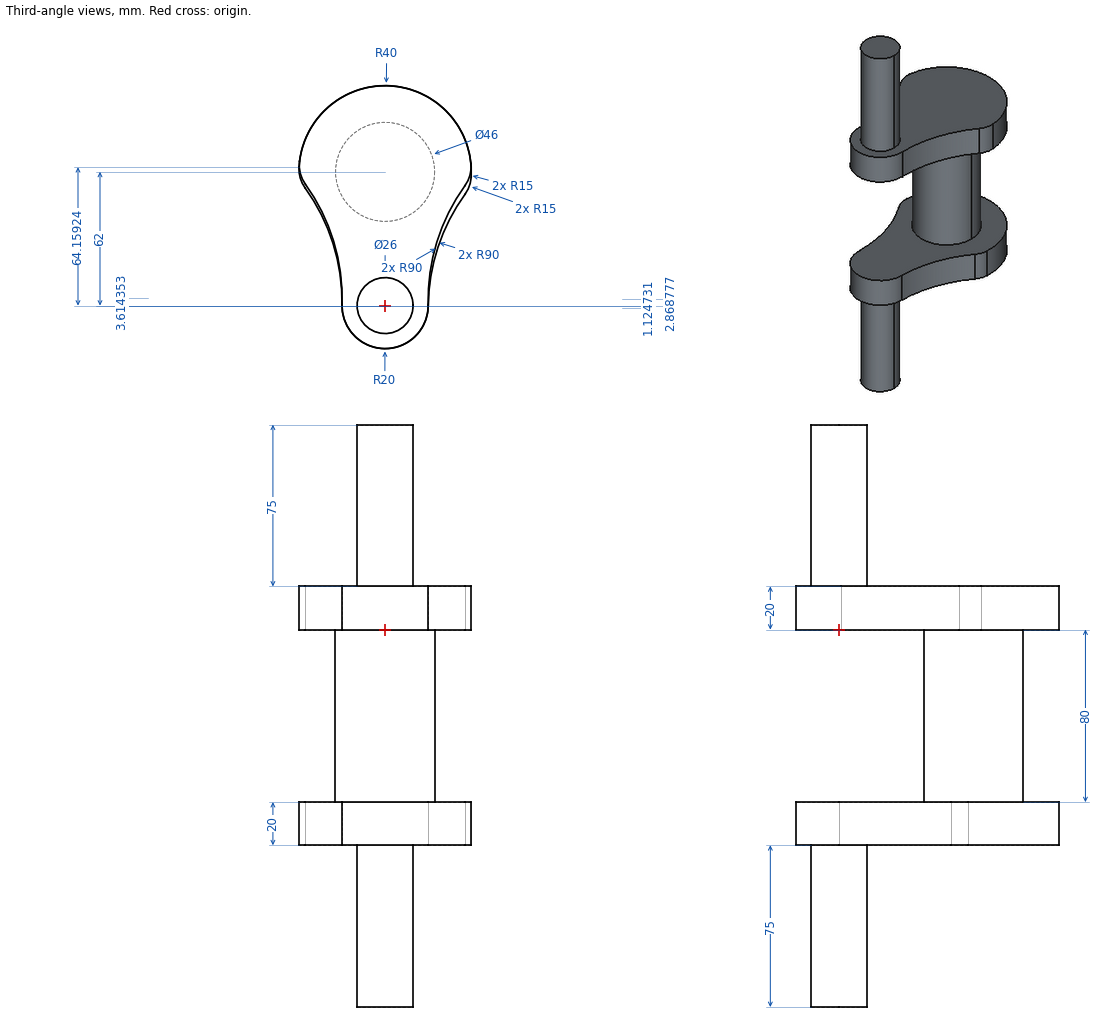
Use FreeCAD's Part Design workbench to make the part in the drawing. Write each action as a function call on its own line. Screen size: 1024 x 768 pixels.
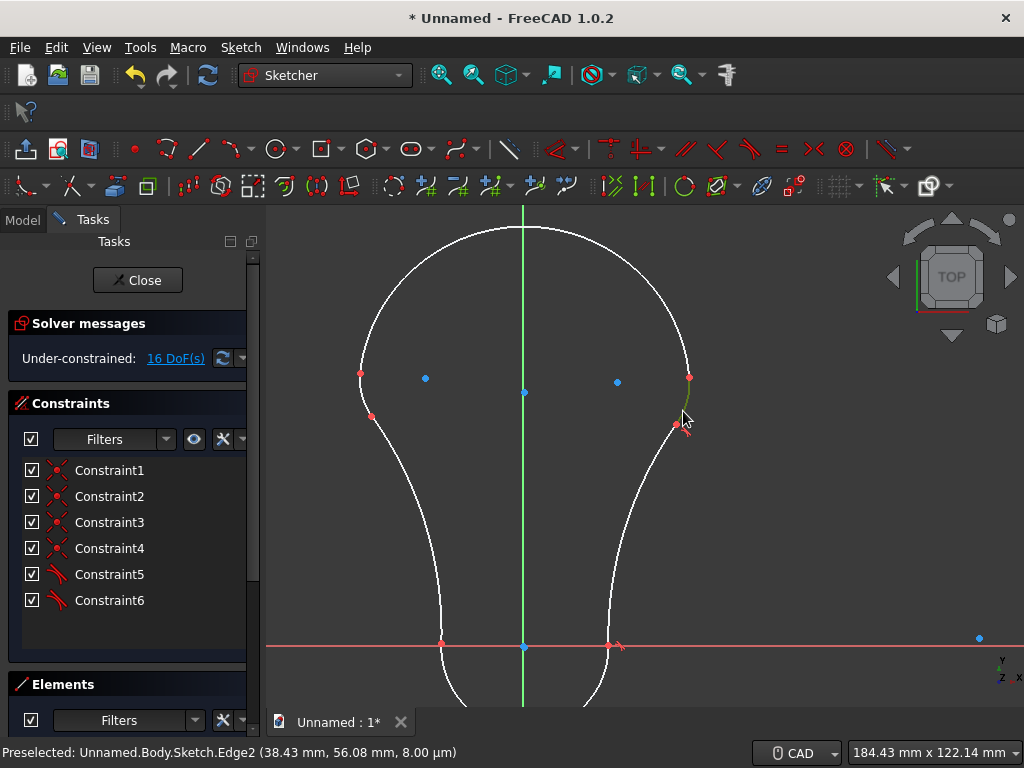
click(618, 256)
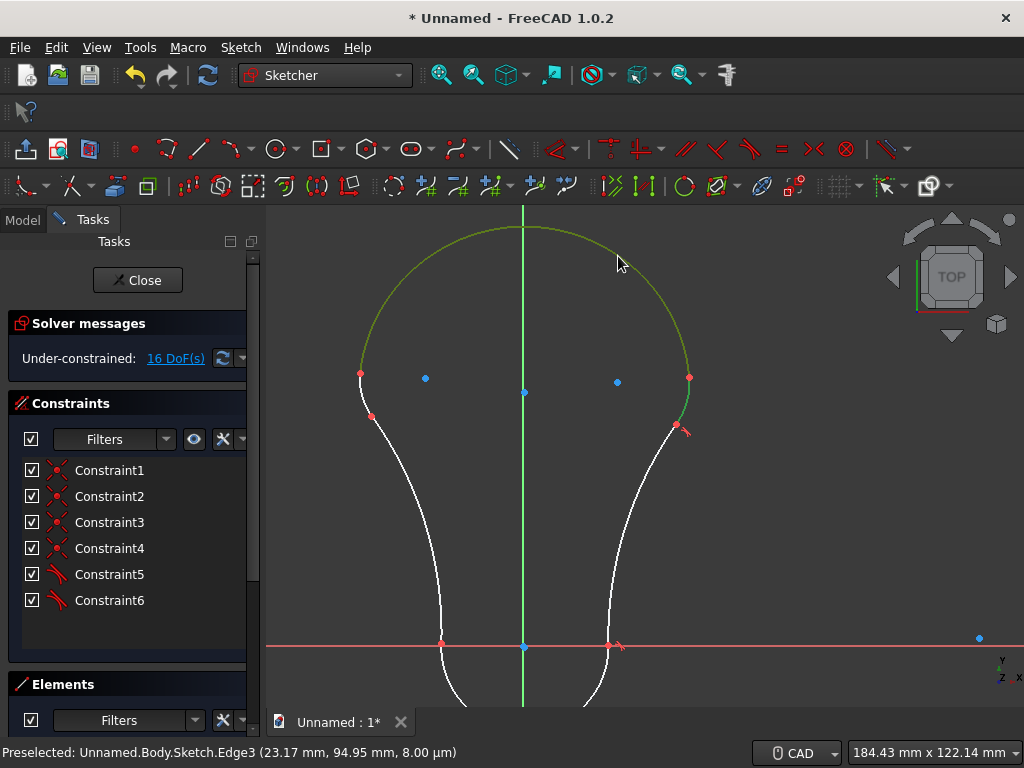
click(750, 150)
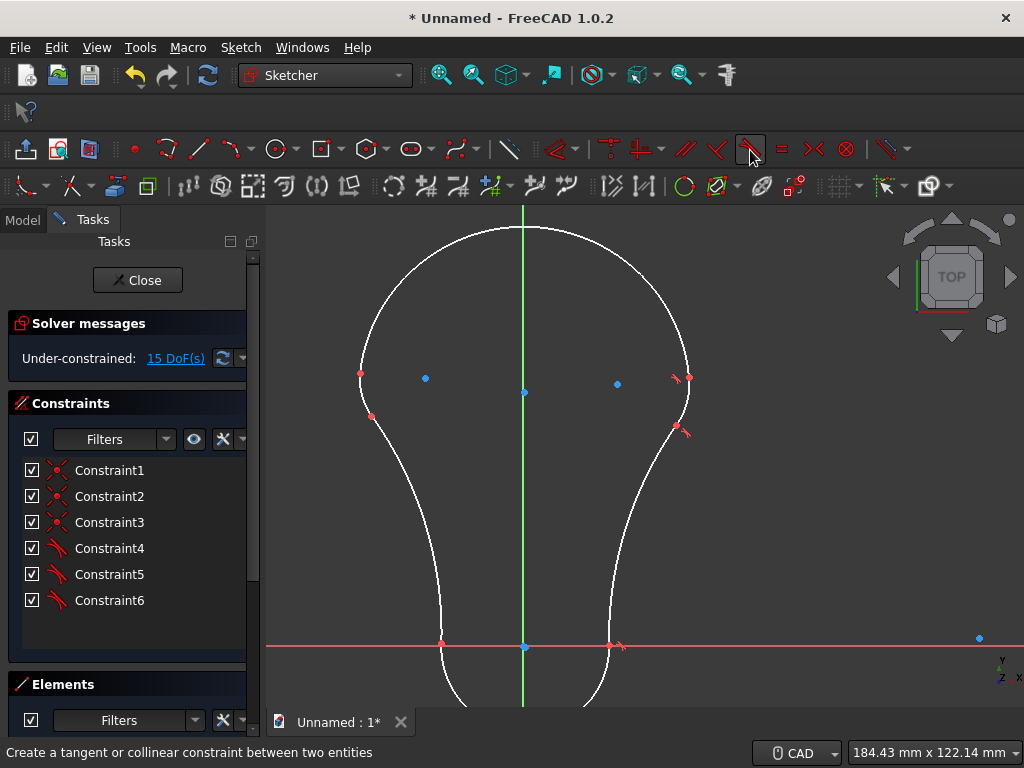
click(618, 256)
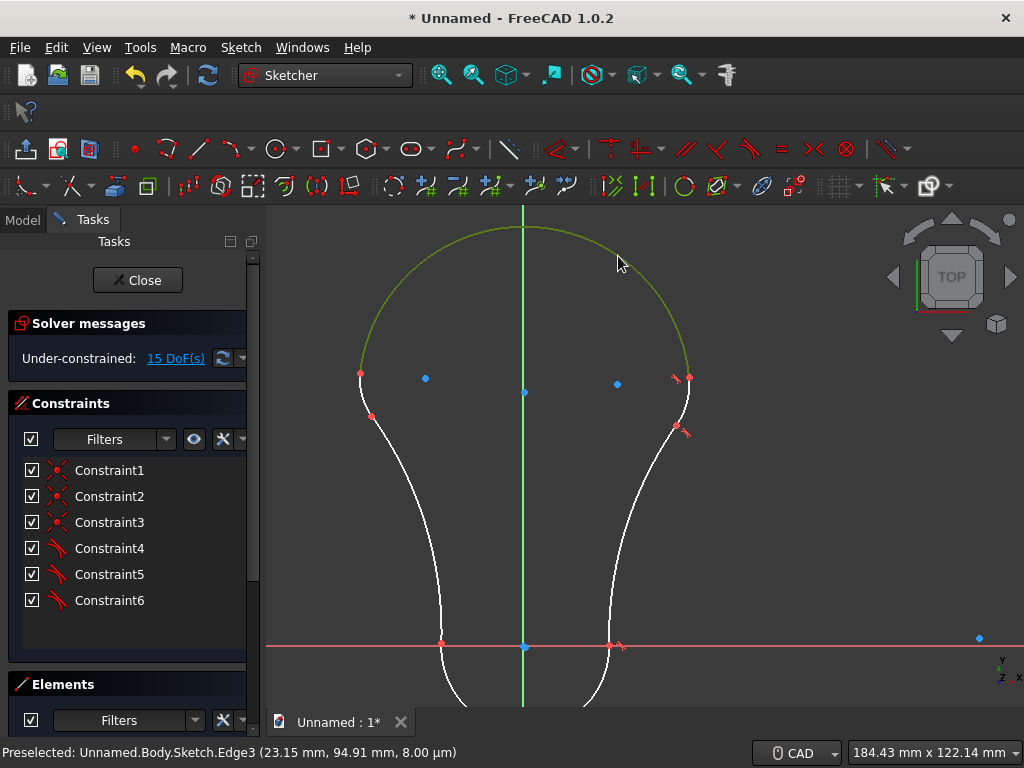
click(360, 387)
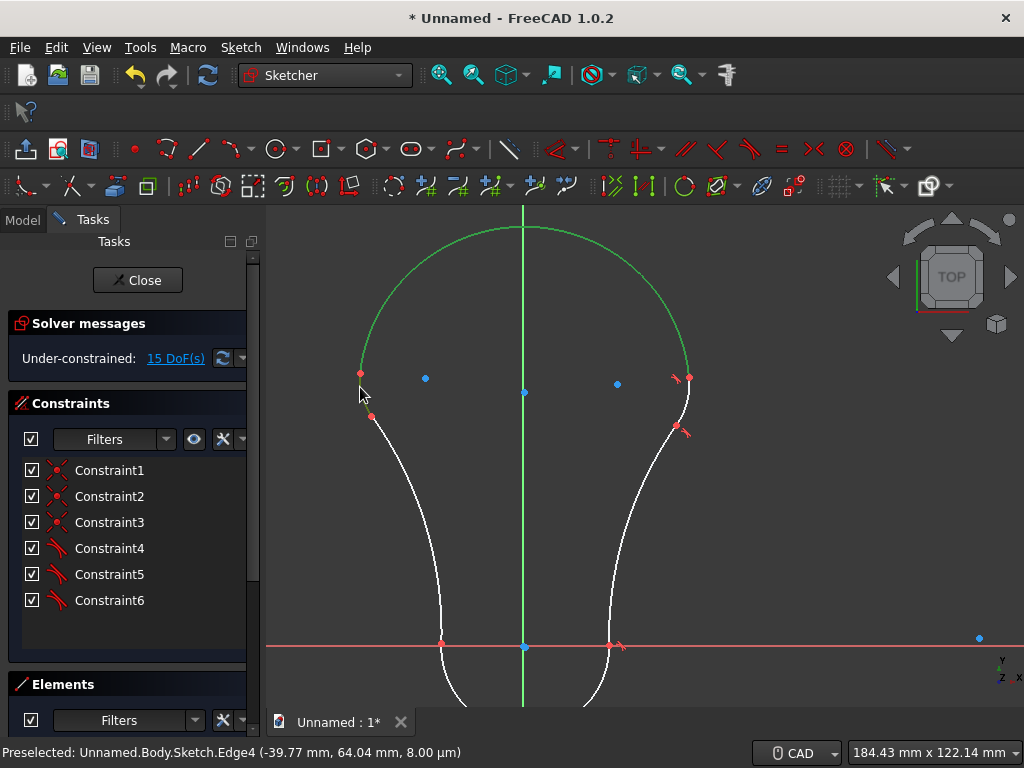
key(t)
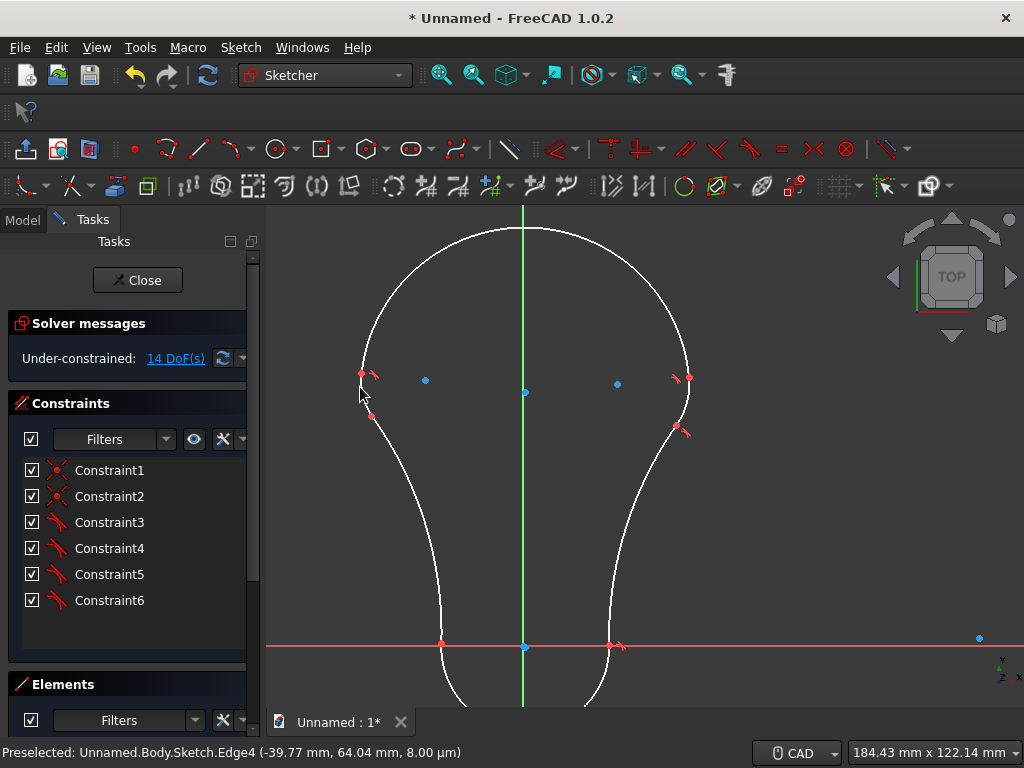
click(361, 387)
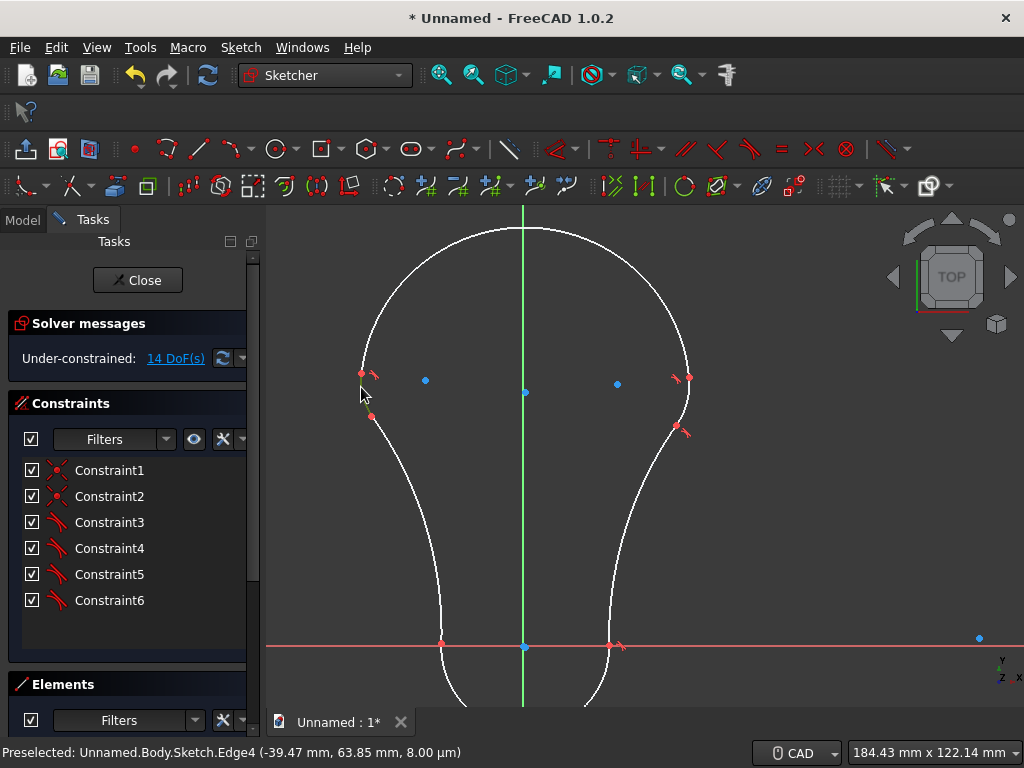
click(436, 571)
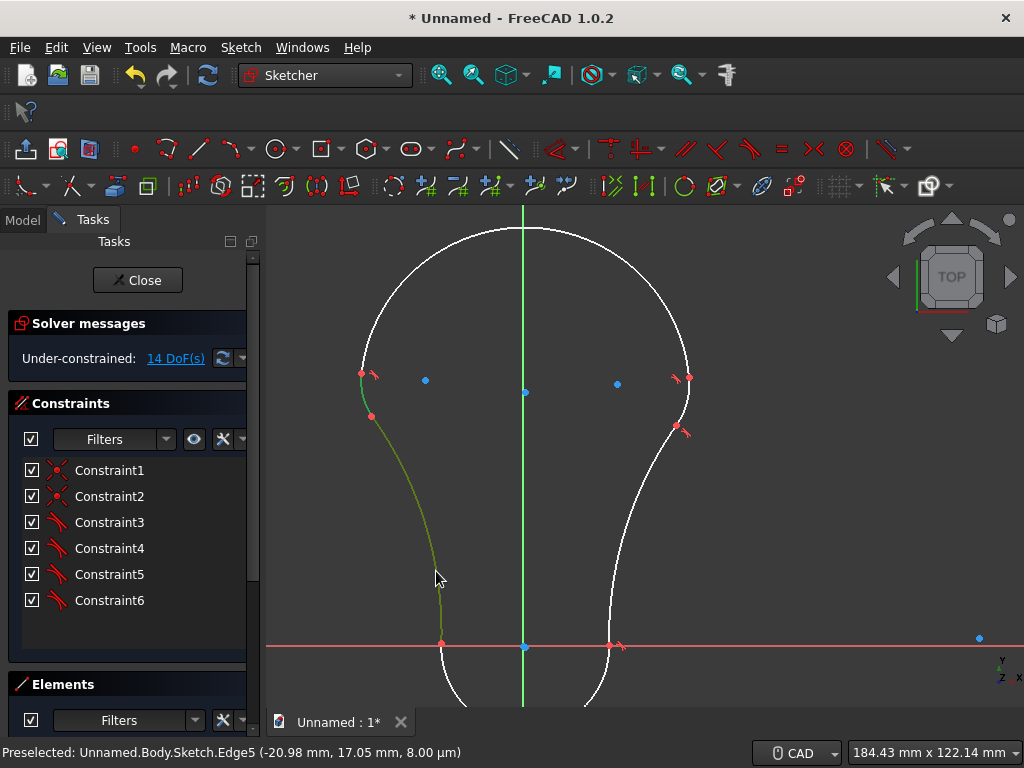
click(750, 150)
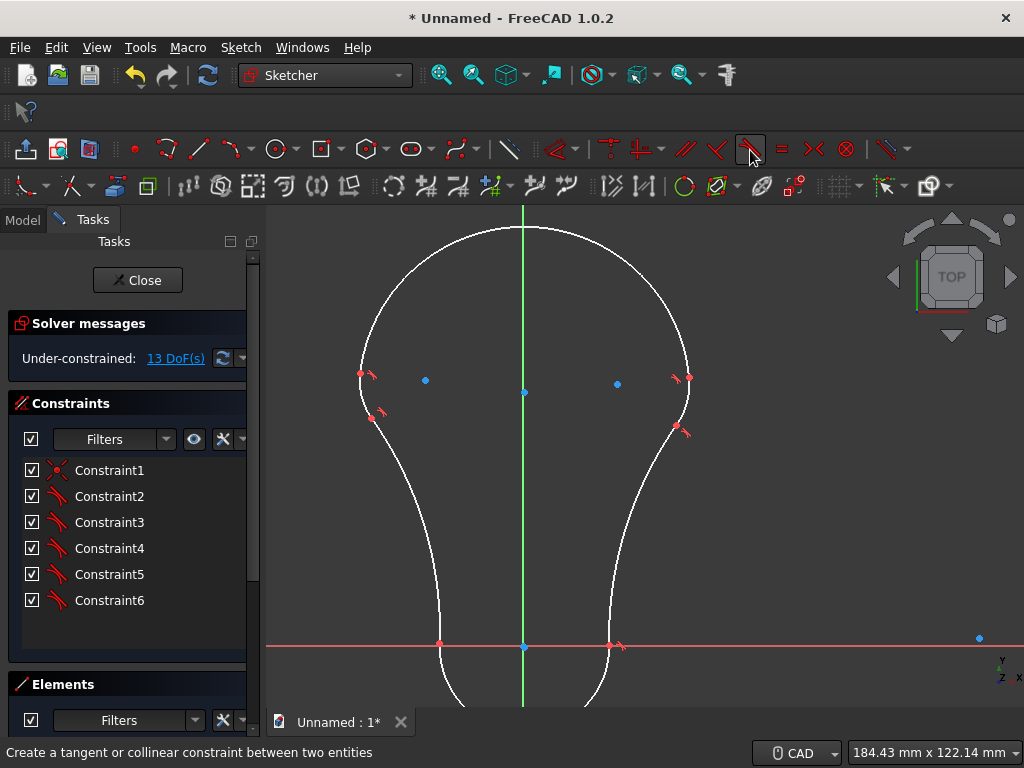
click(435, 572)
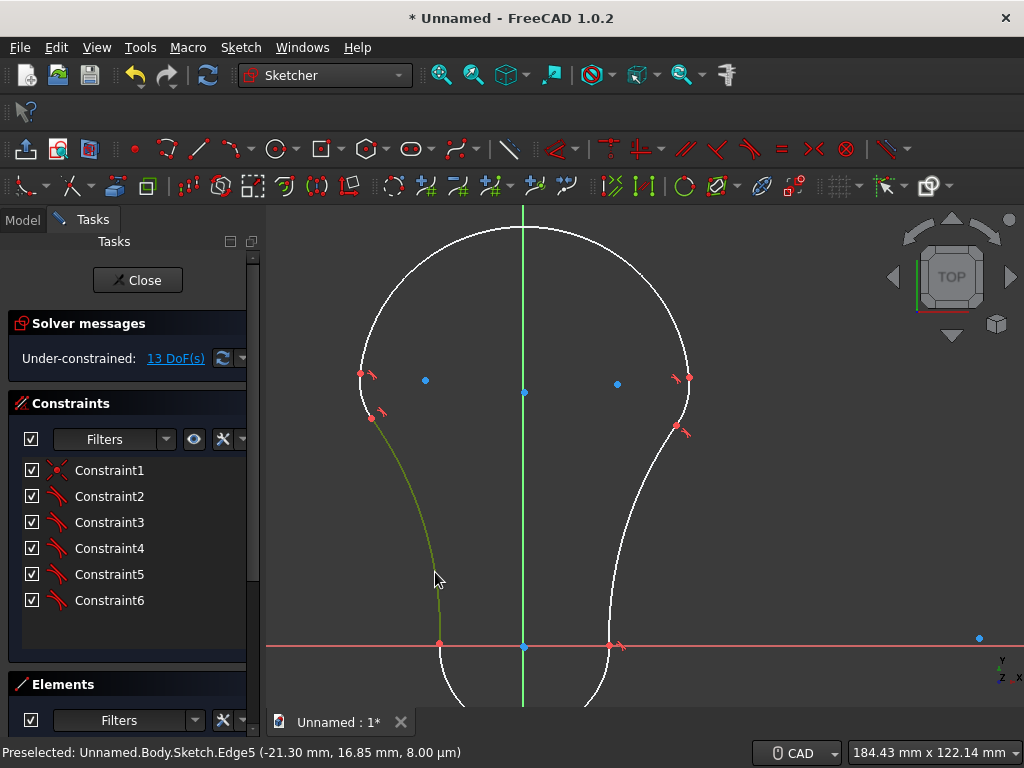
scroll(684, 412, down, 2)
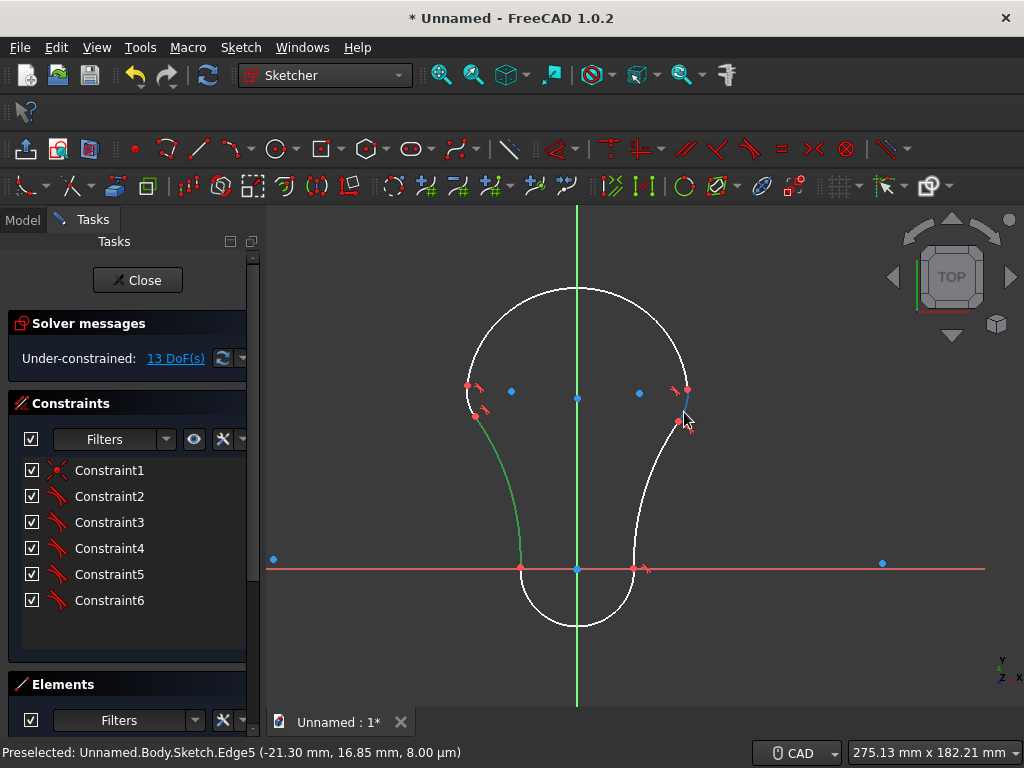
click(543, 615)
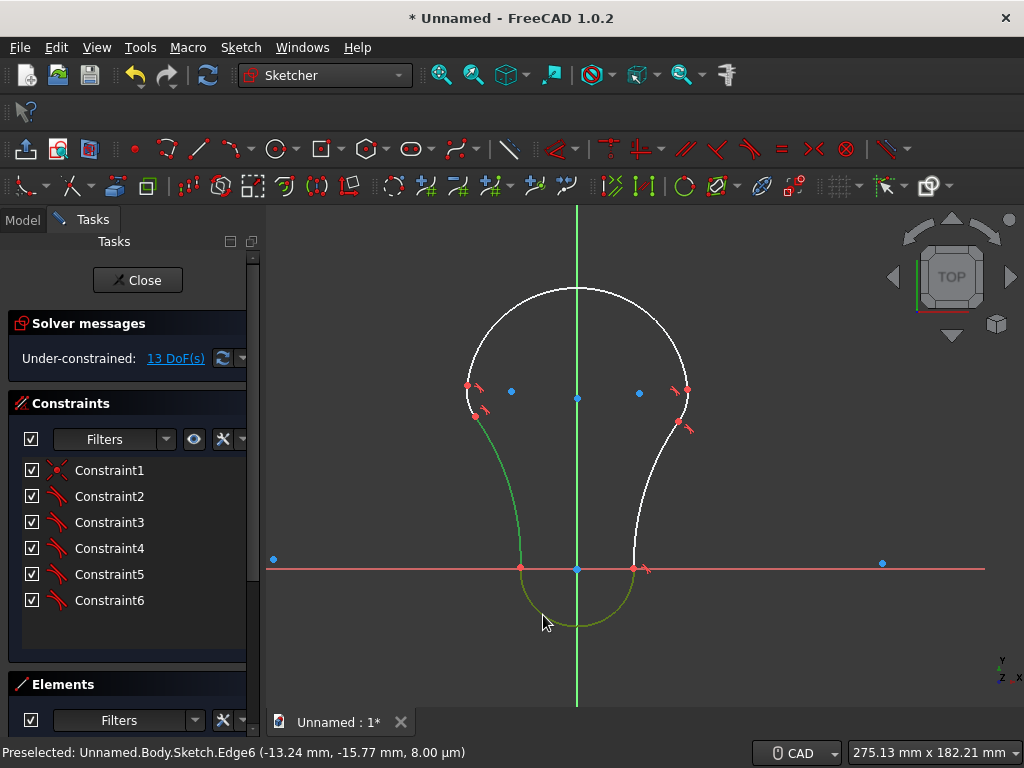
click(750, 150)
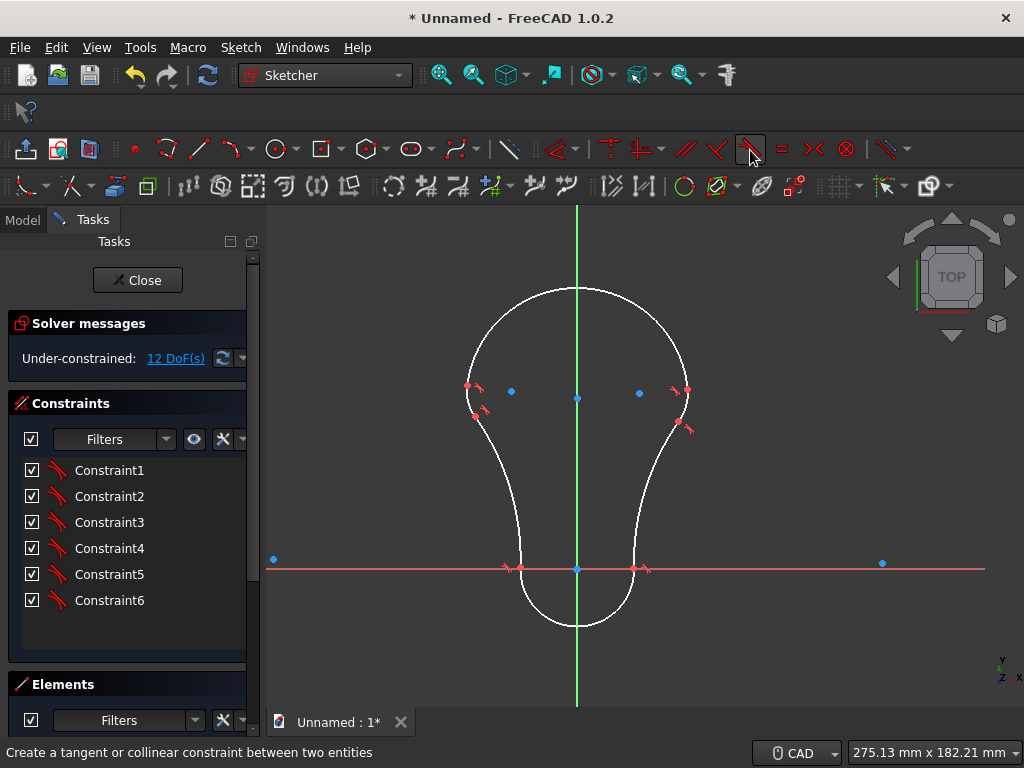
drag(567, 559, 587, 580)